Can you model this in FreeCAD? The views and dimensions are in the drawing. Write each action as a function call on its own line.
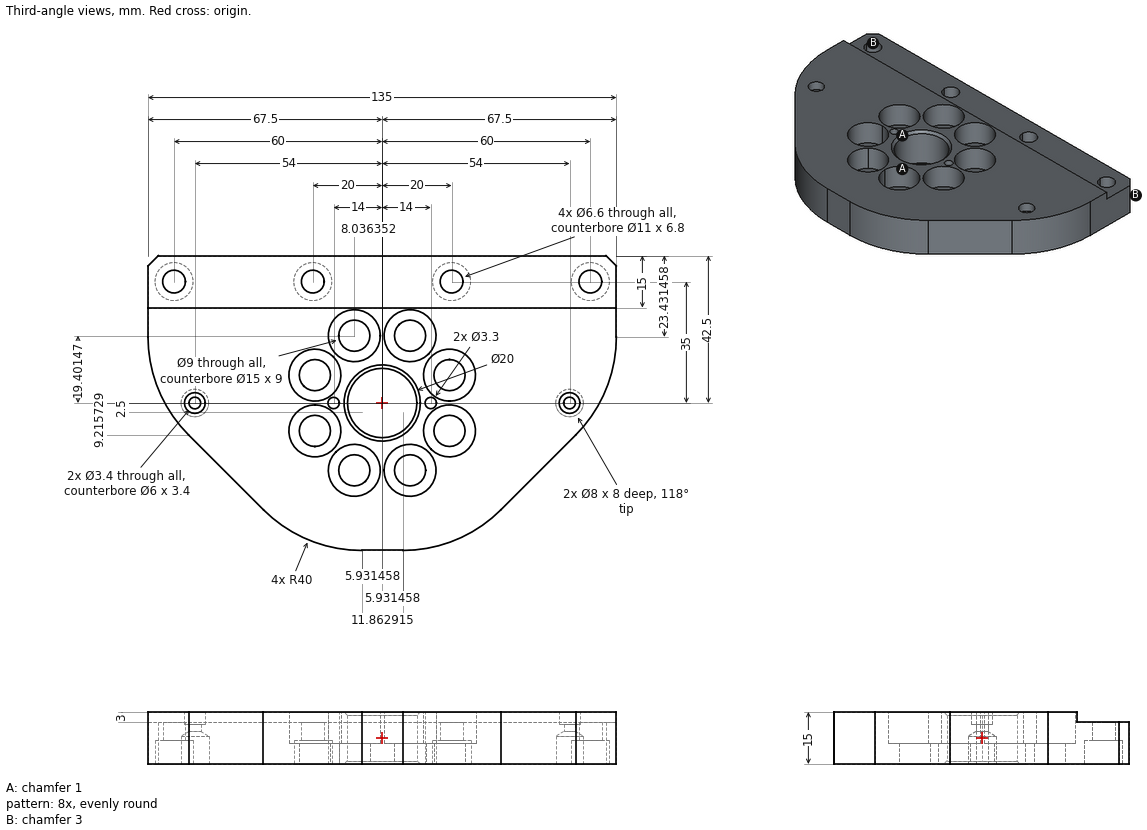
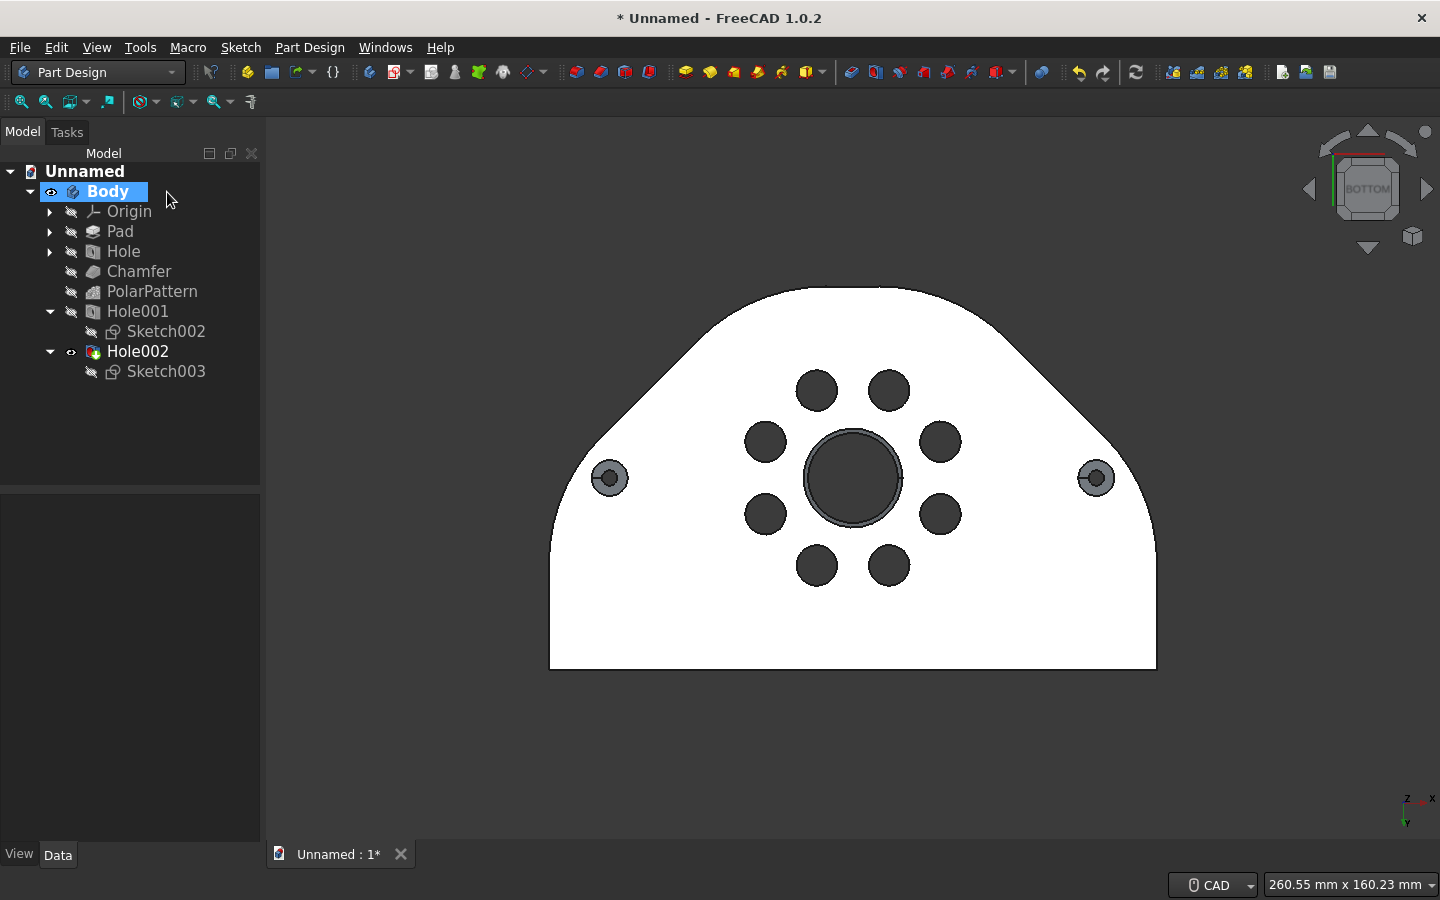
click(1027, 586)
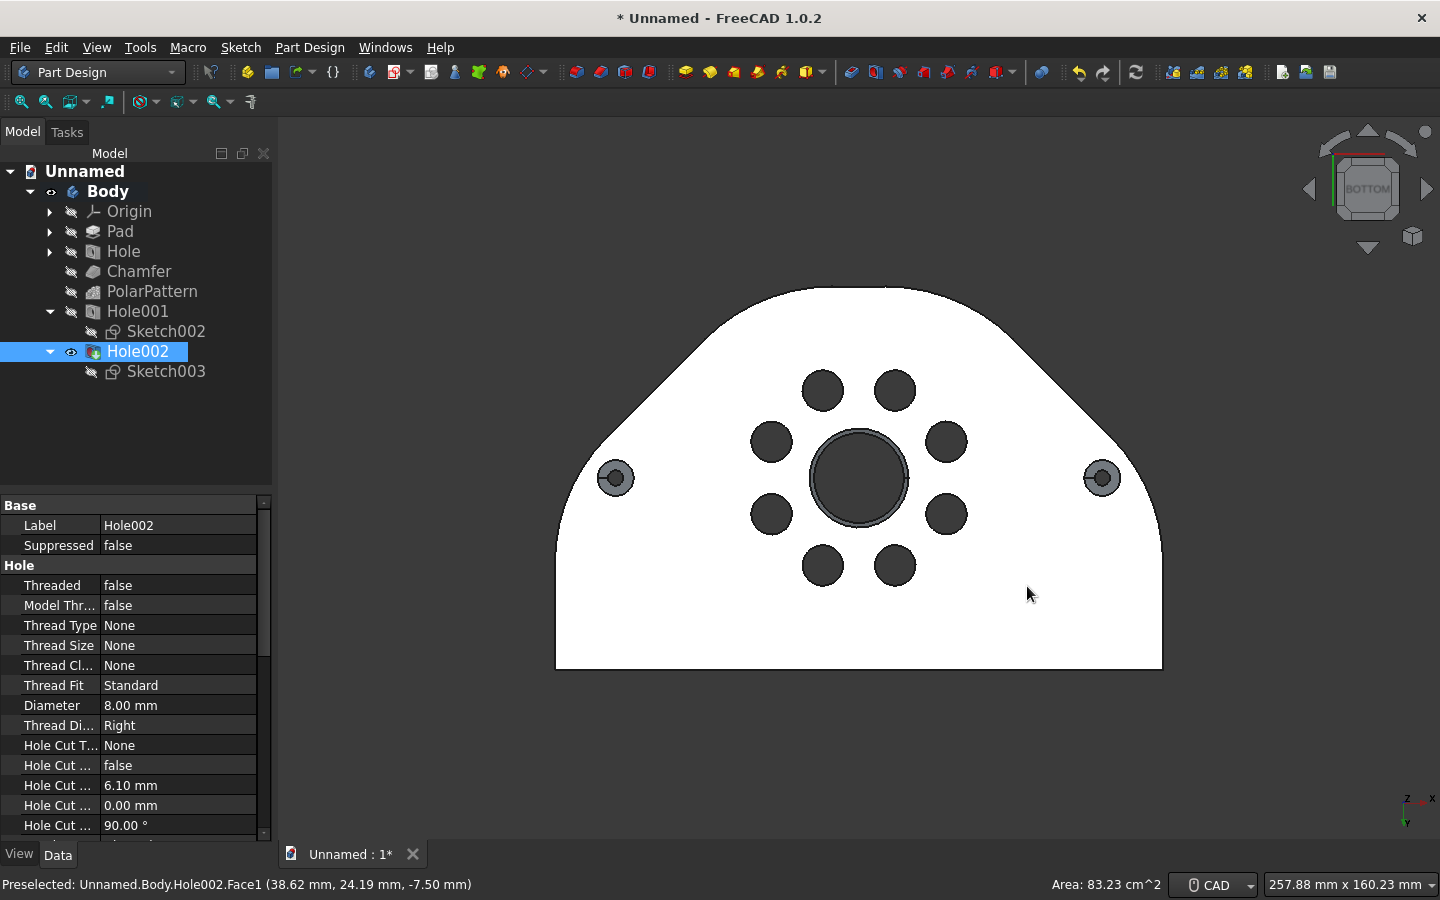
click(394, 72)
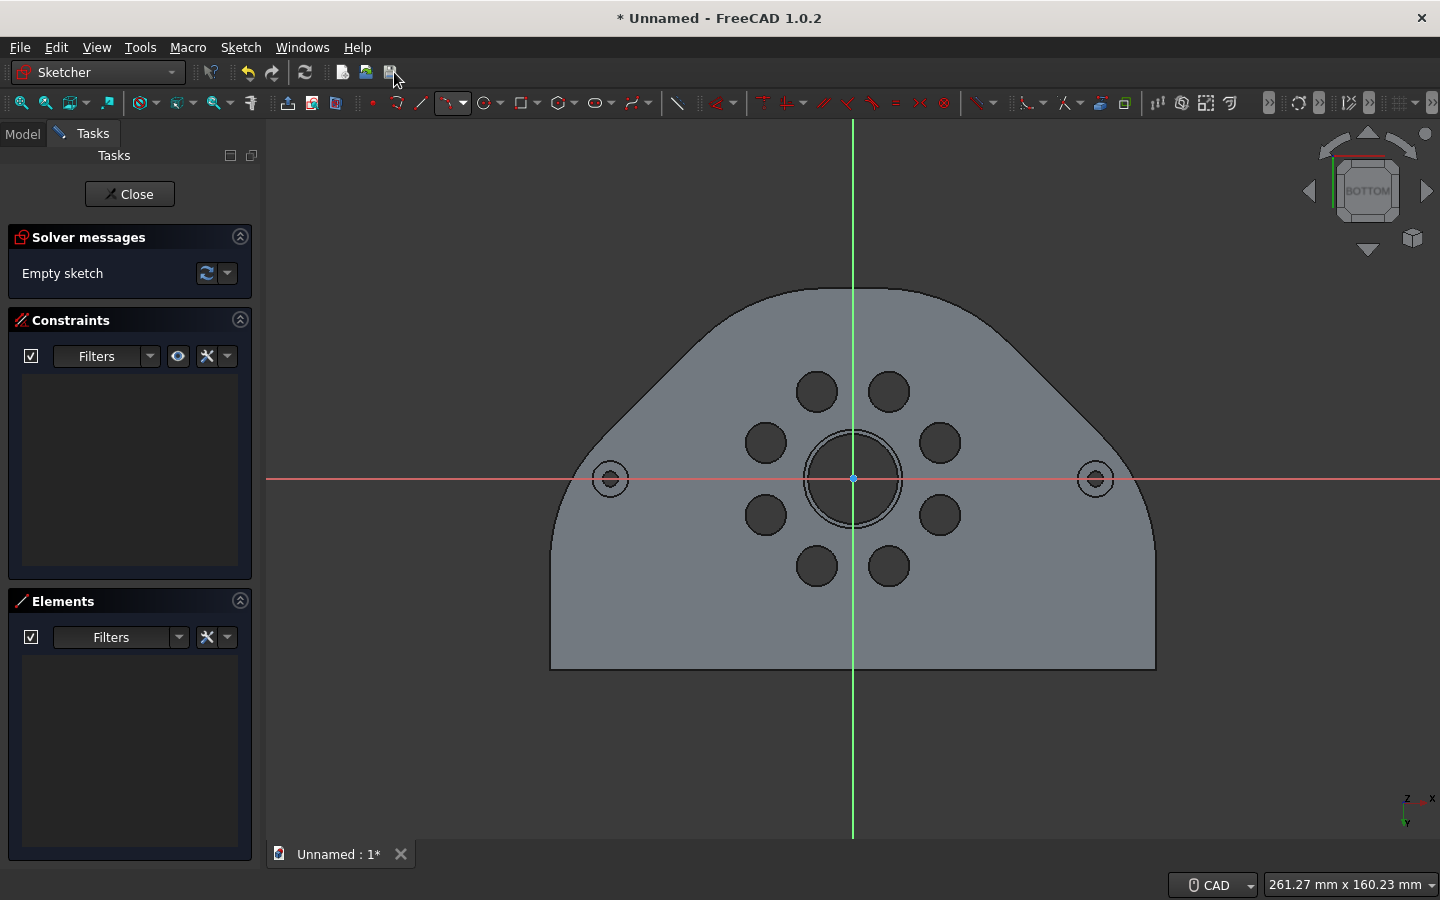
scroll(870, 479, up, 8)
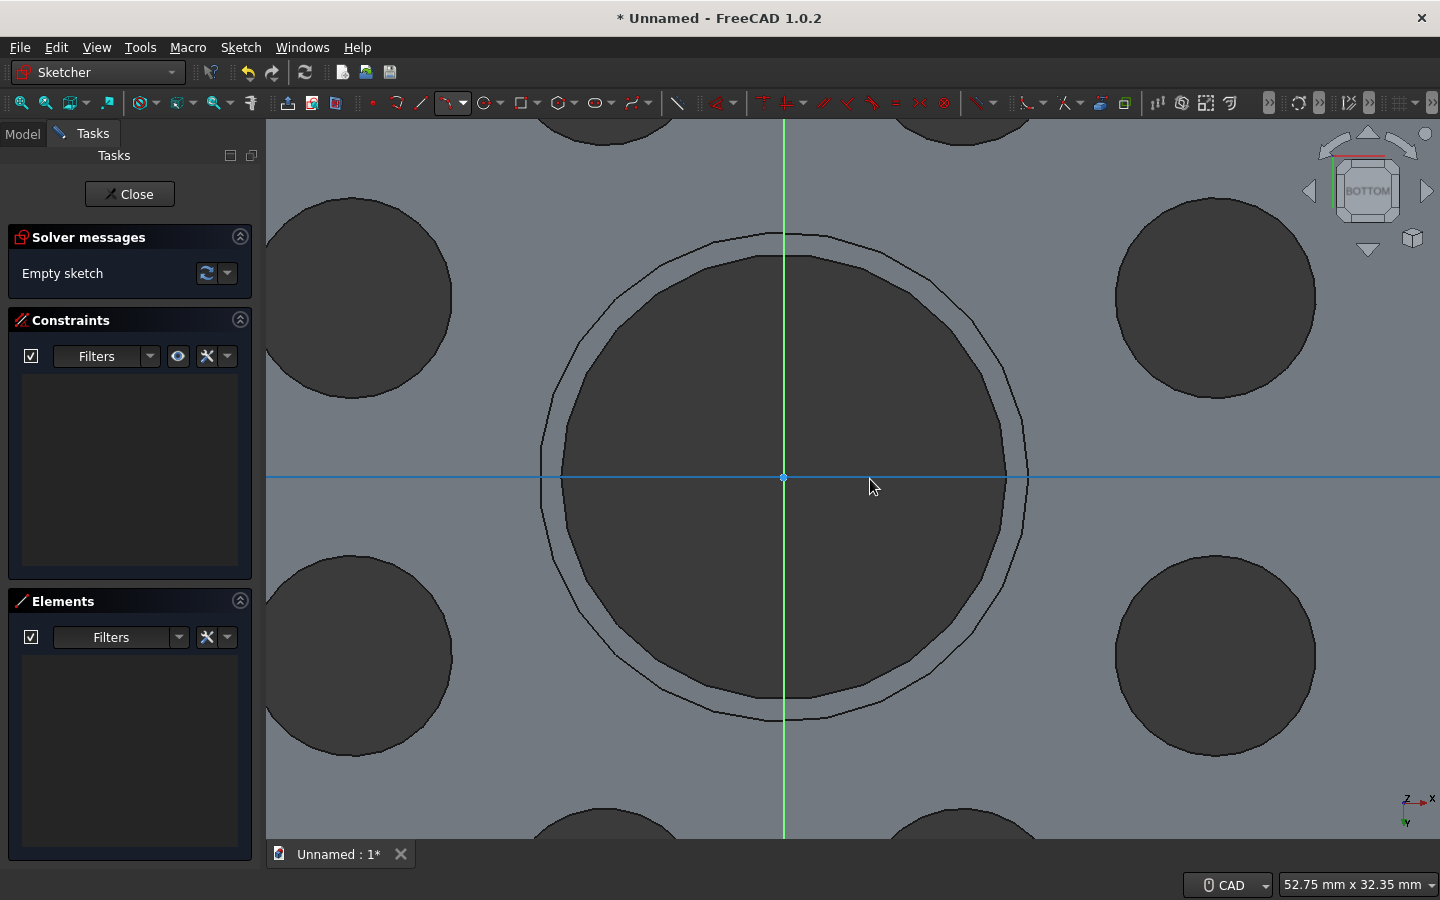
click(484, 104)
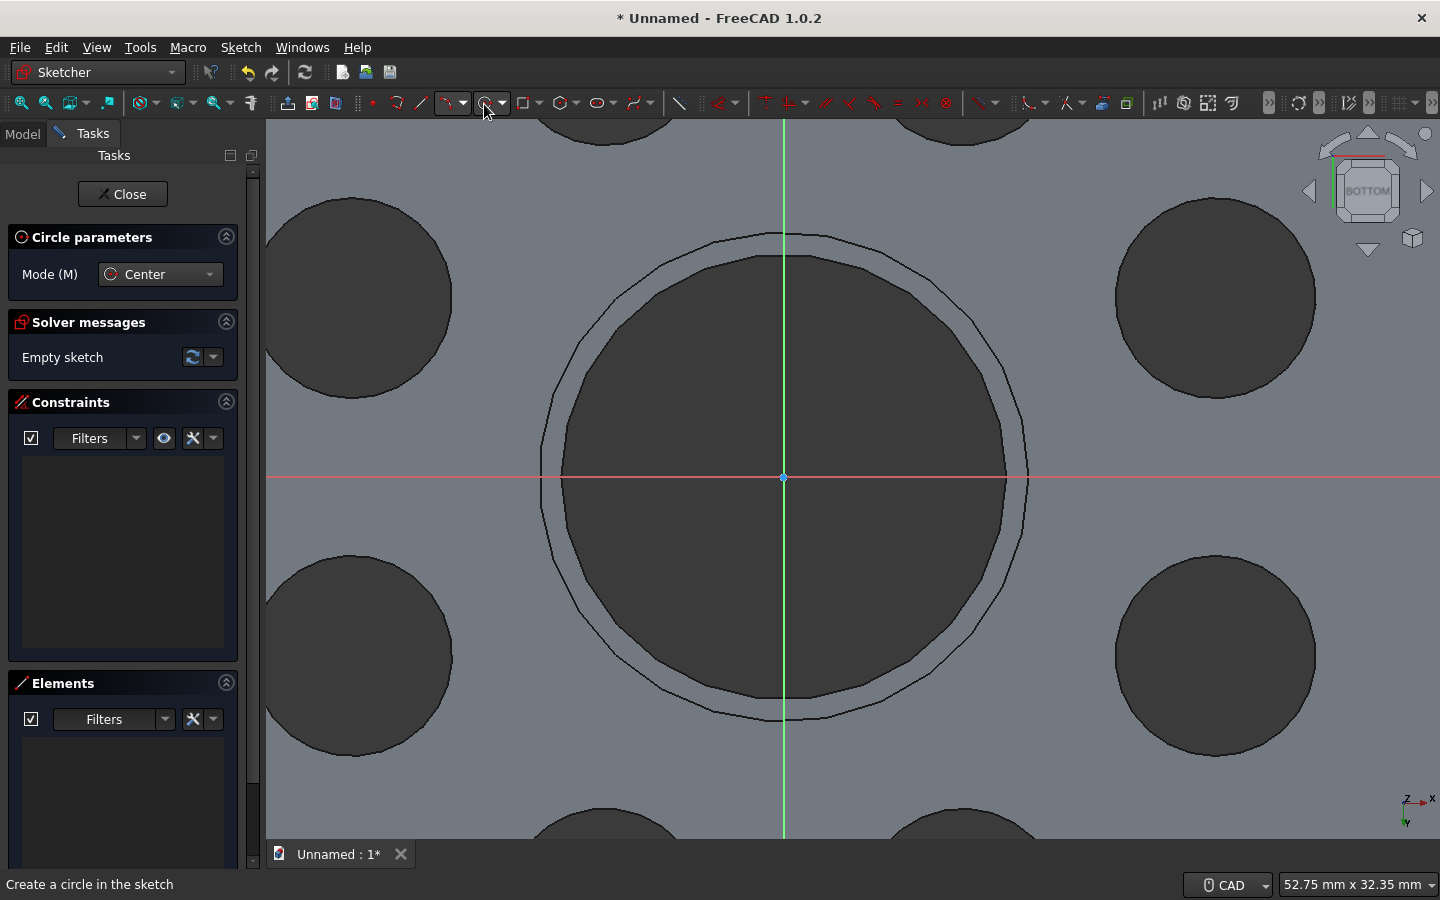
click(1095, 477)
move(1121, 451)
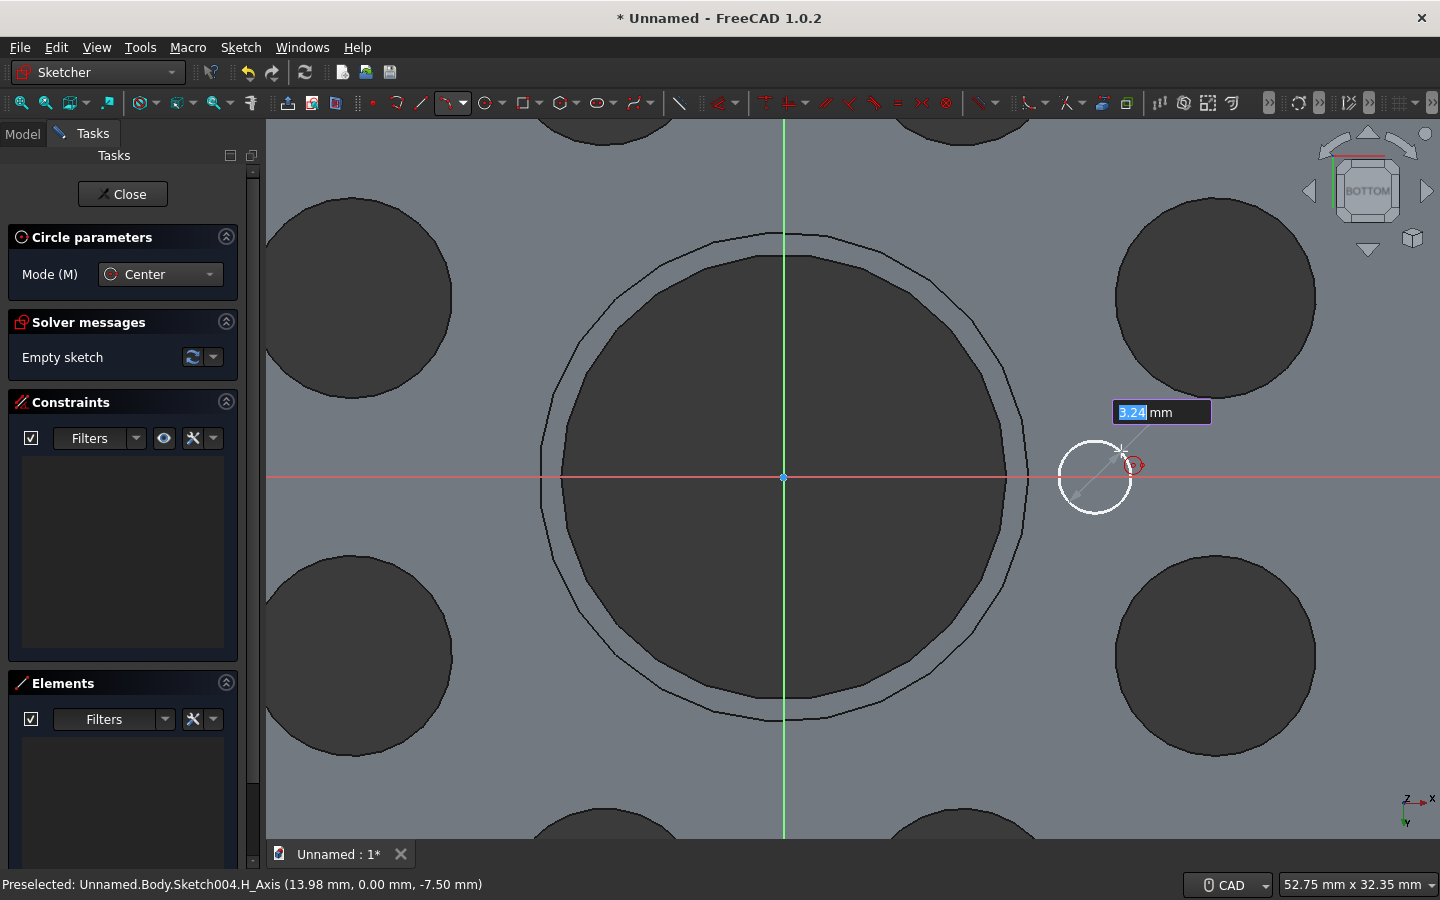
text(3.3)
key(Return)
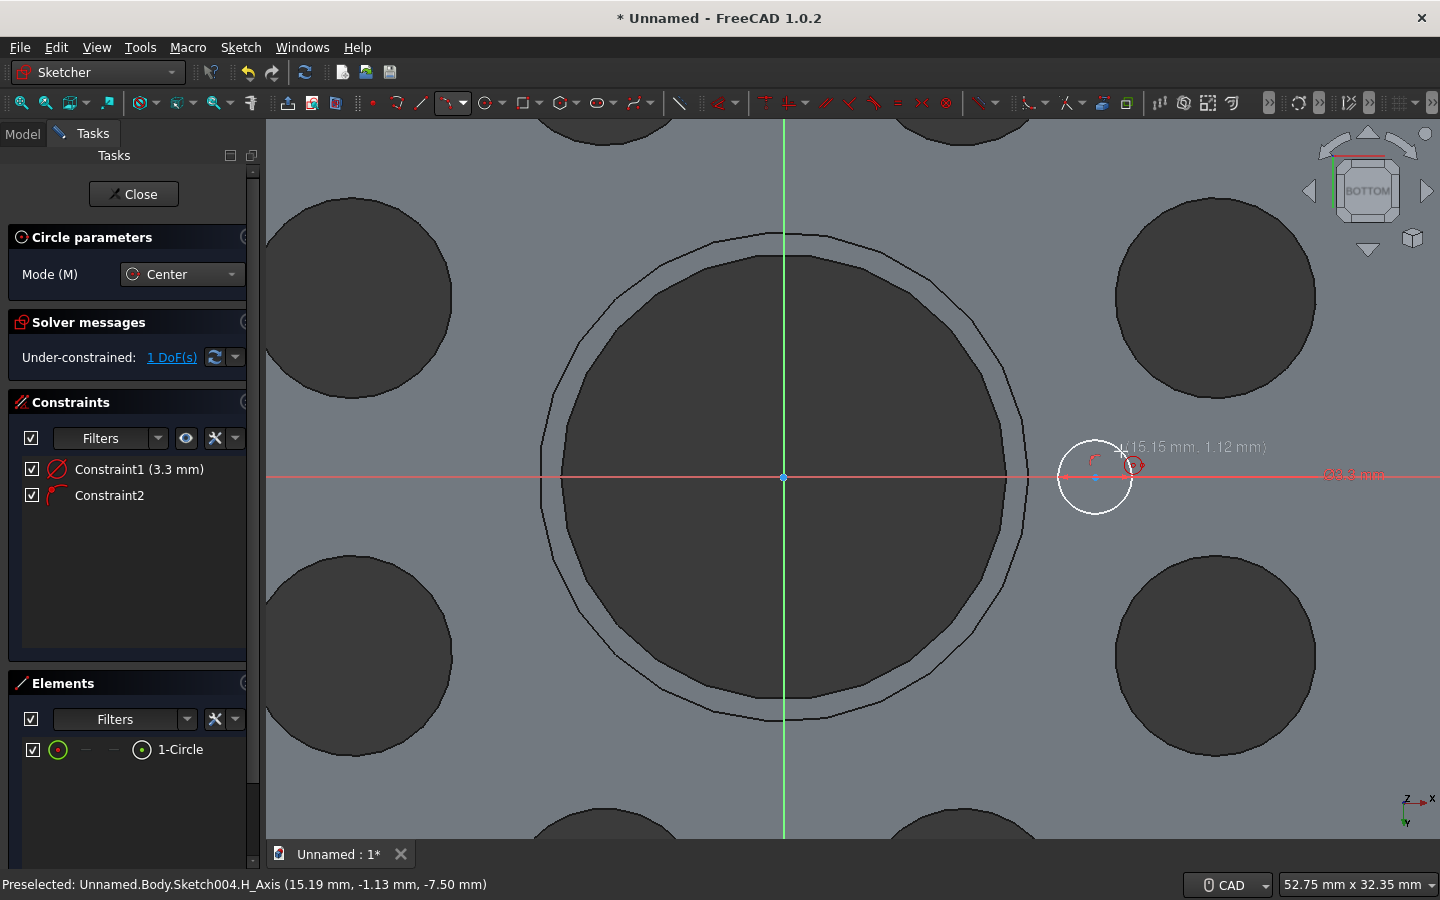
click(472, 477)
move(498, 451)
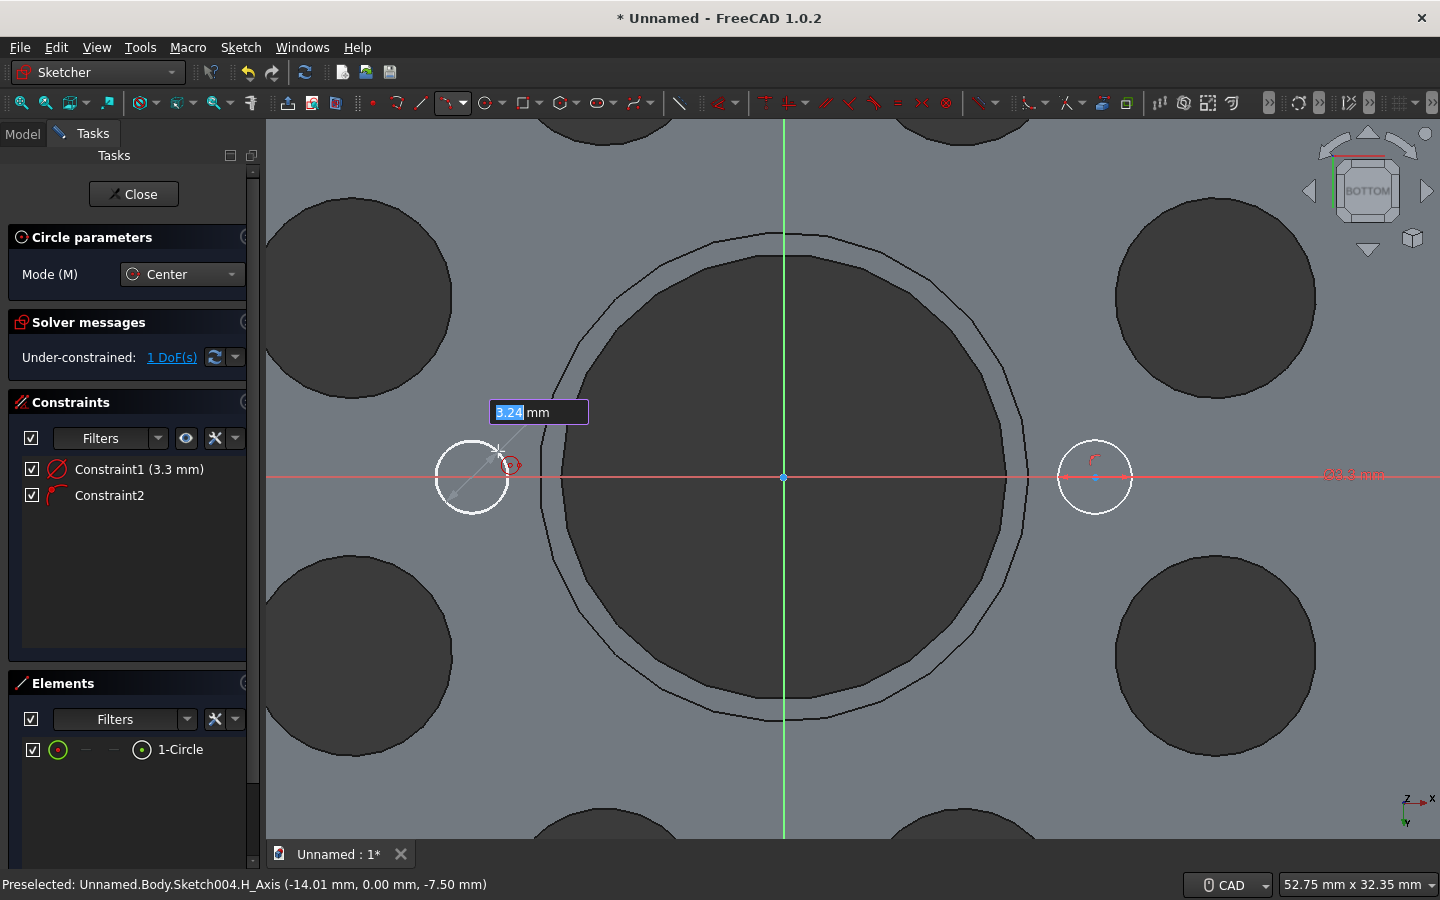
text(3.3)
key(Return)
key(Escape)